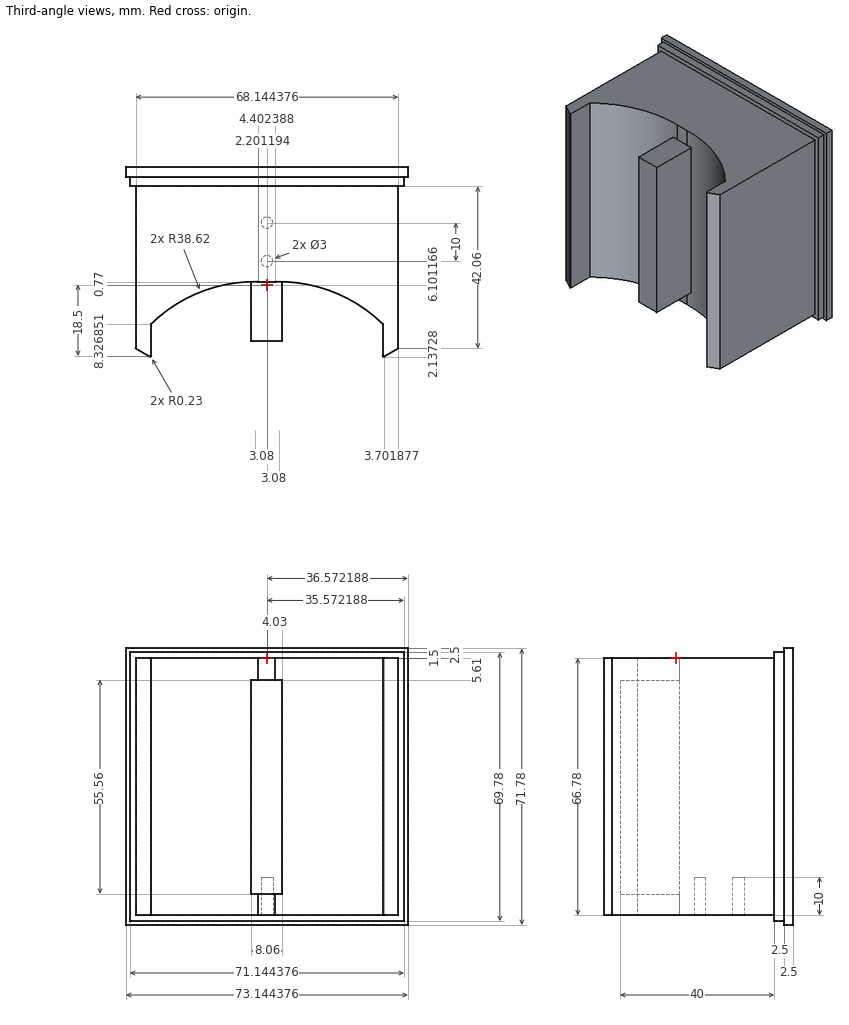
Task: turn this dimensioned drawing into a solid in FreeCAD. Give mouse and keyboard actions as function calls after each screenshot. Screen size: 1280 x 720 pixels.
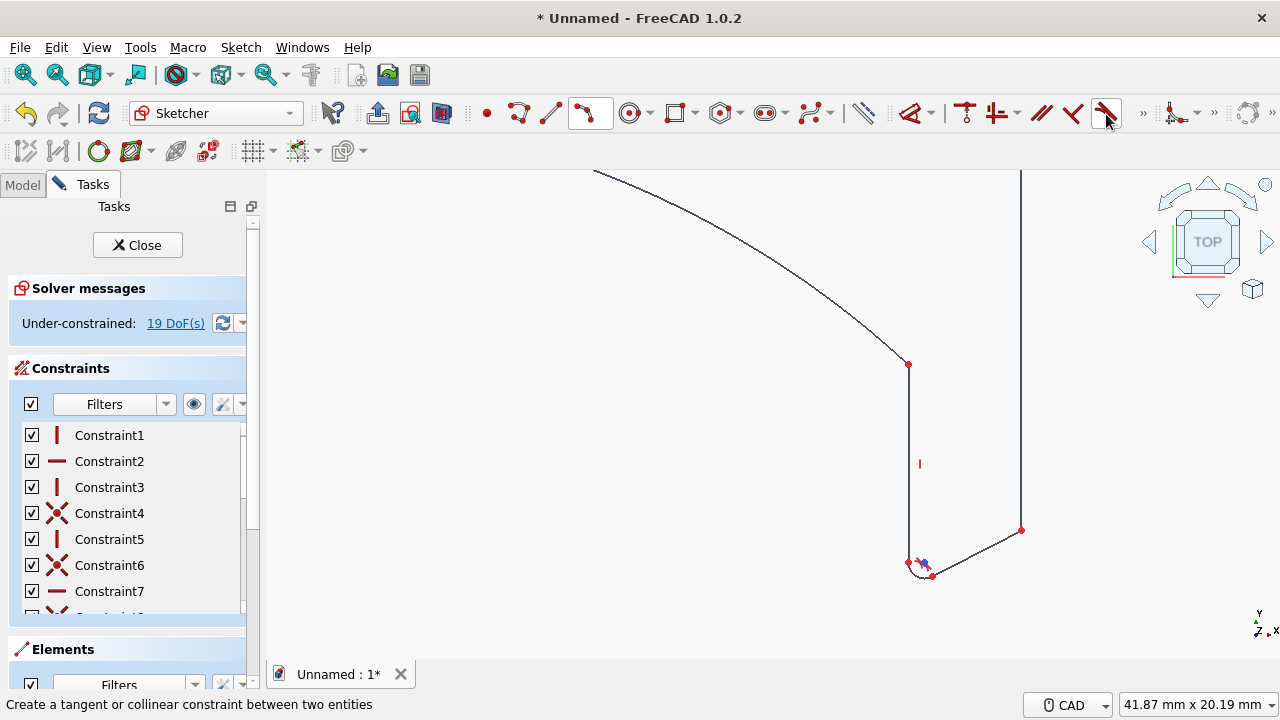
scroll(924, 575, down, 6)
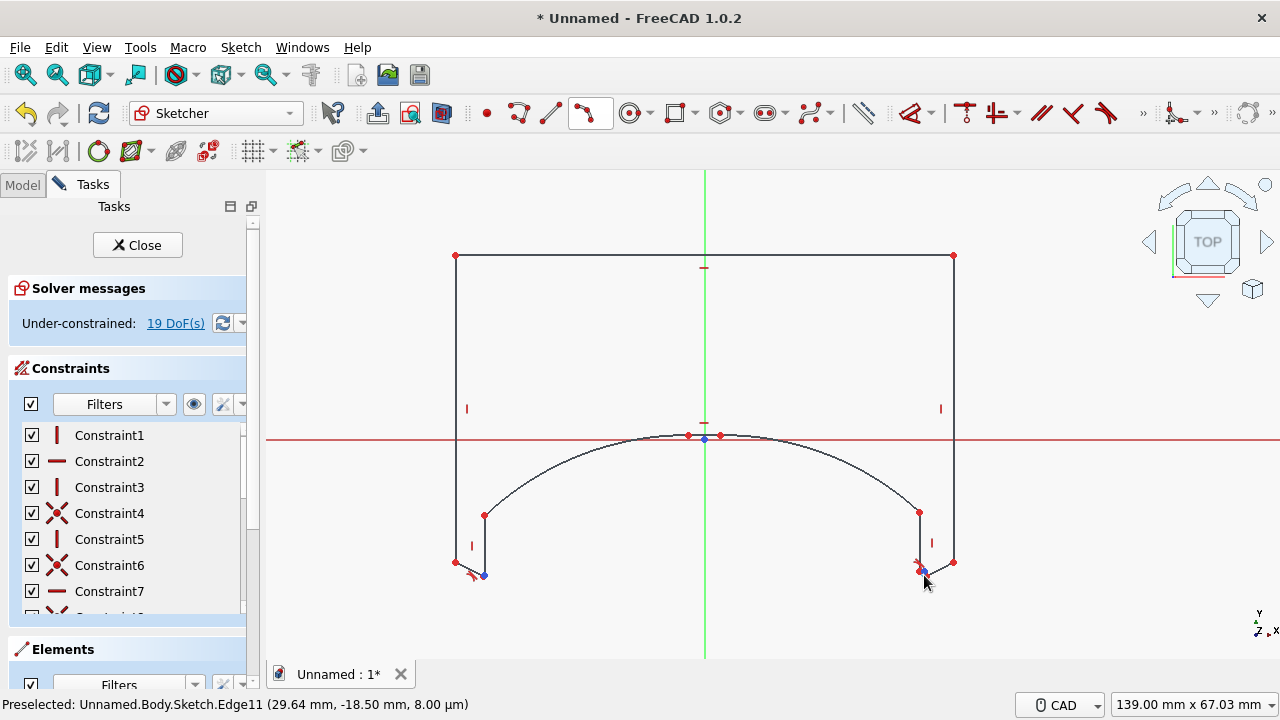
scroll(464, 566, up, 2)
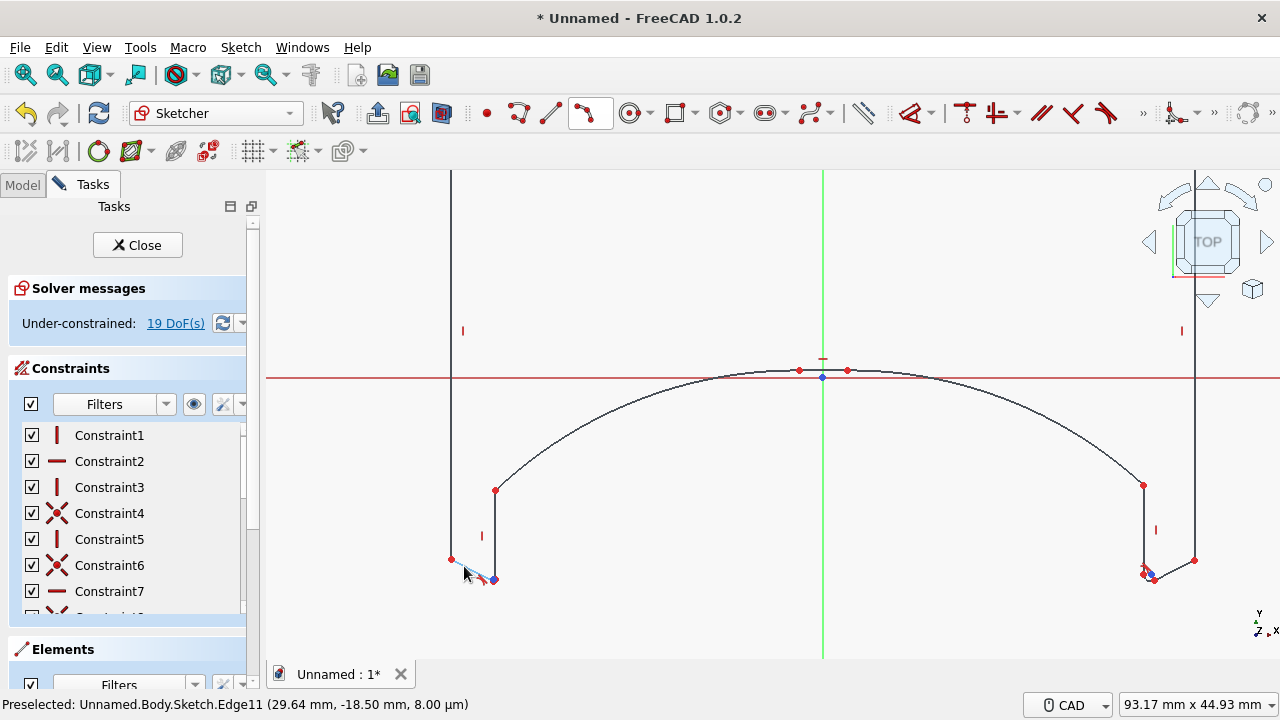
click(464, 566)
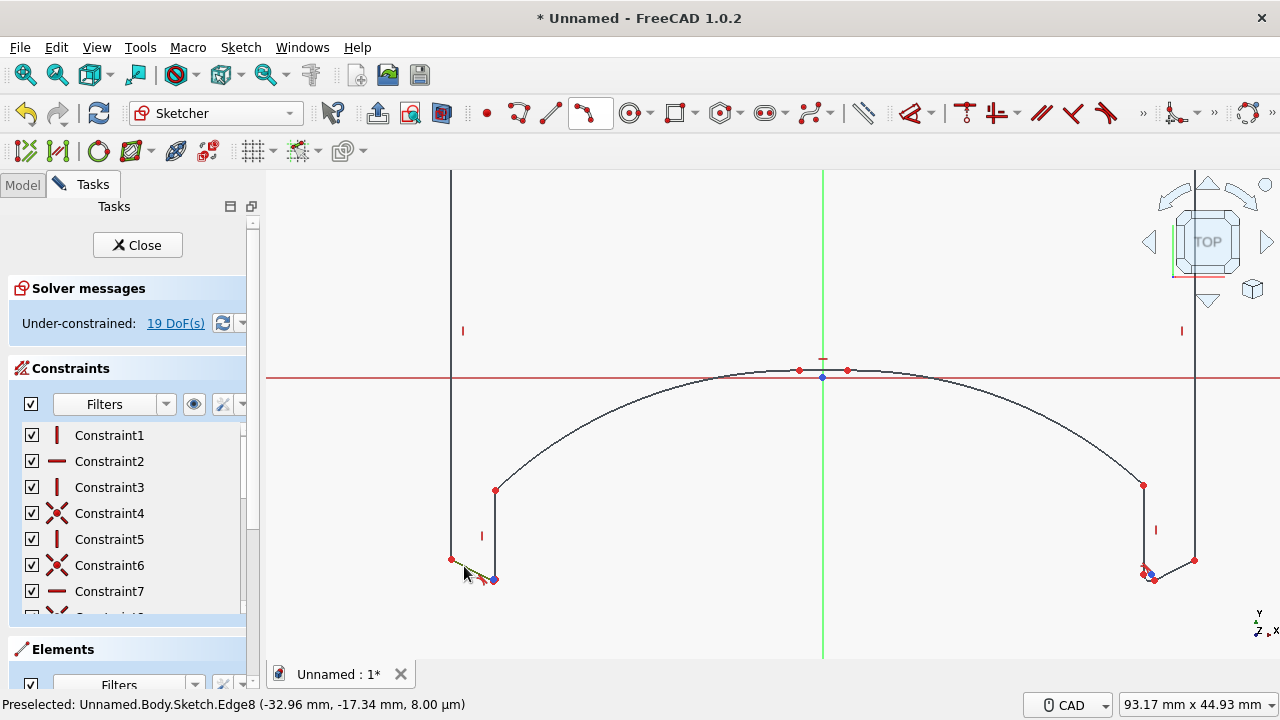
scroll(495, 581, up, 12)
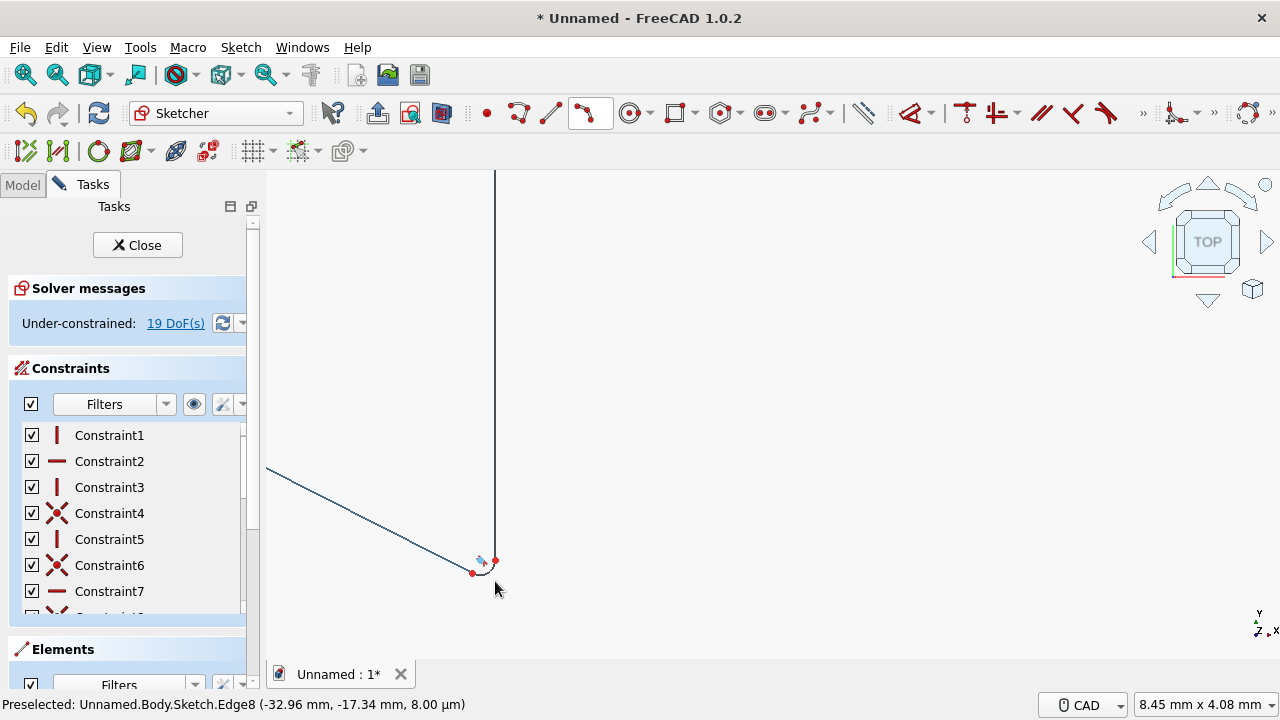
click(488, 573)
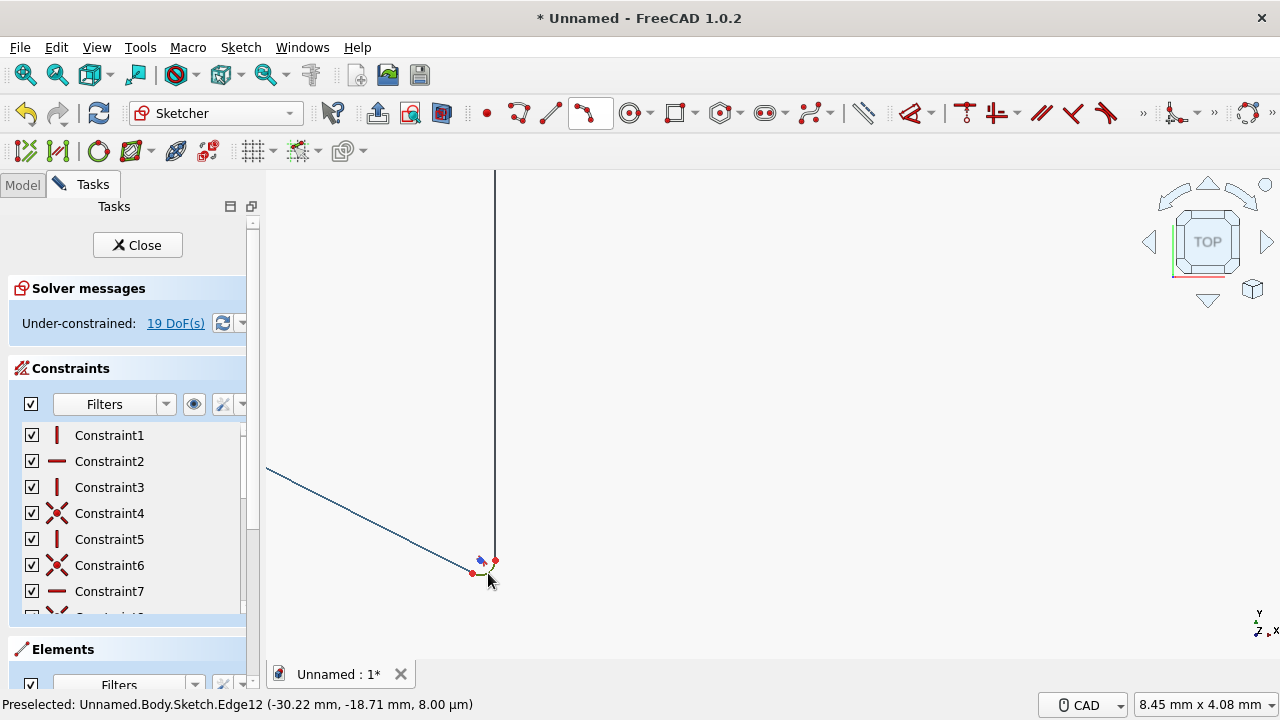
click(1106, 114)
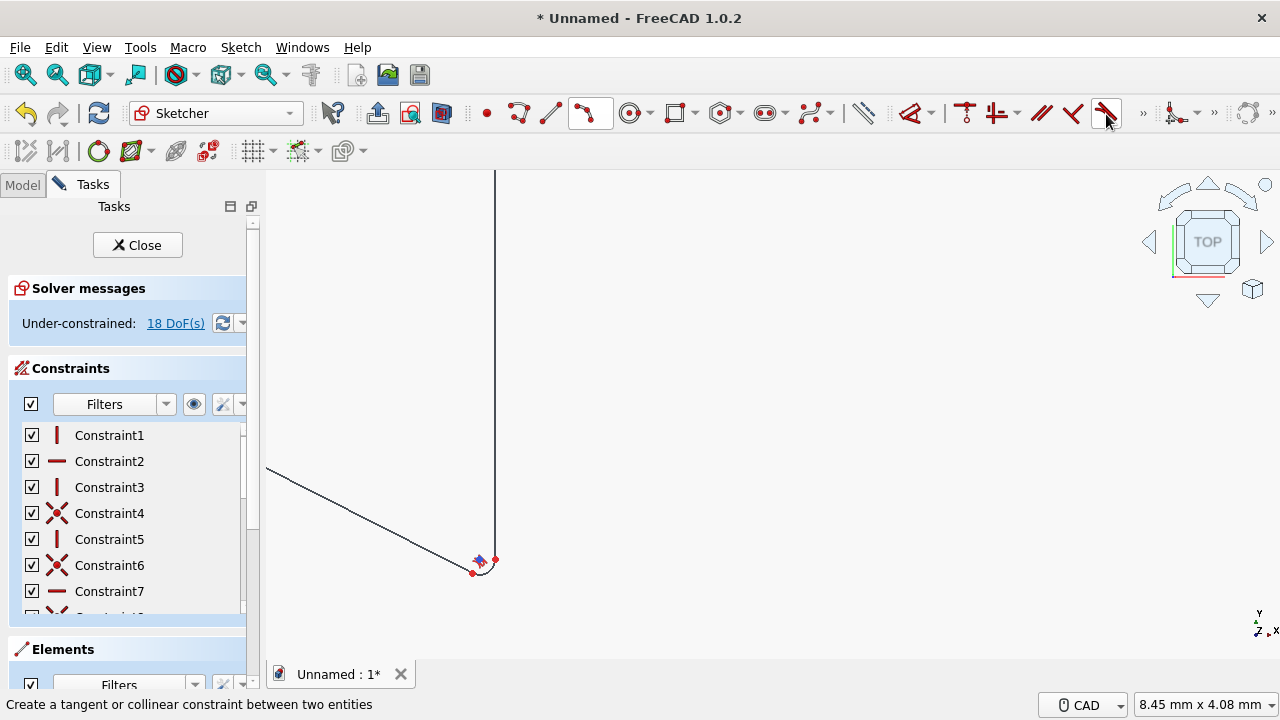
scroll(484, 576, down, 14)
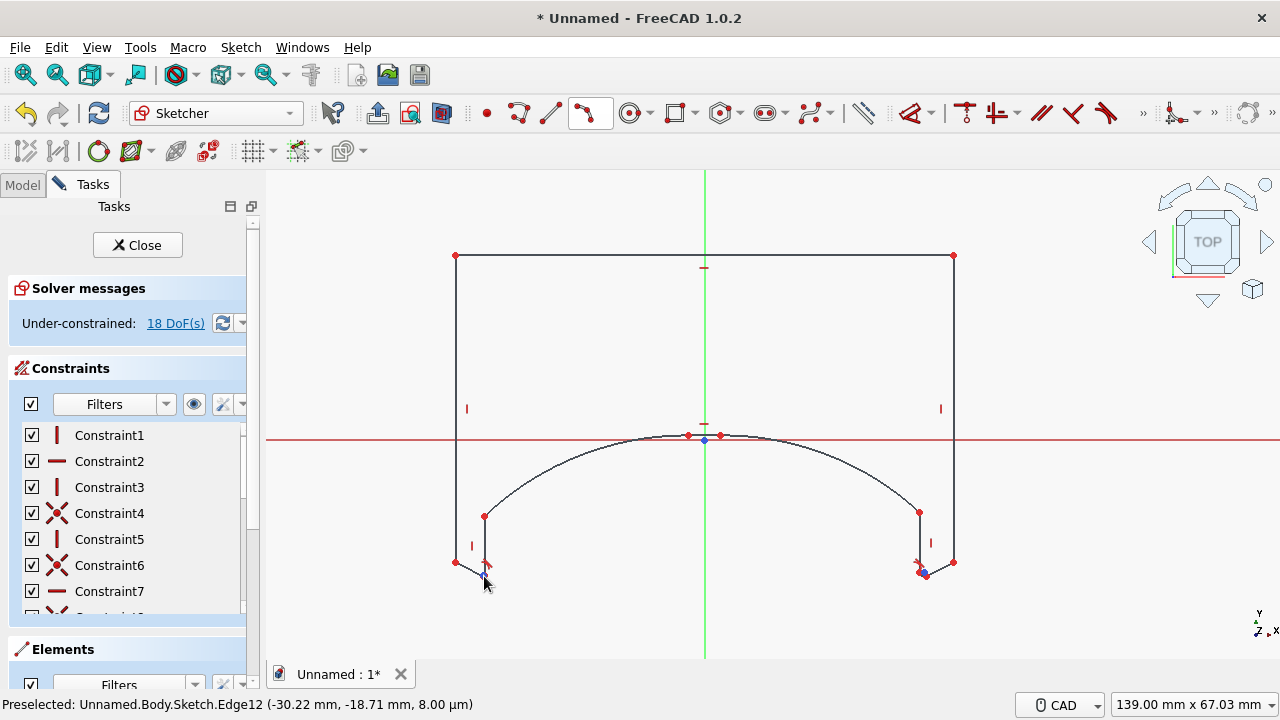
scroll(622, 443, up, 9)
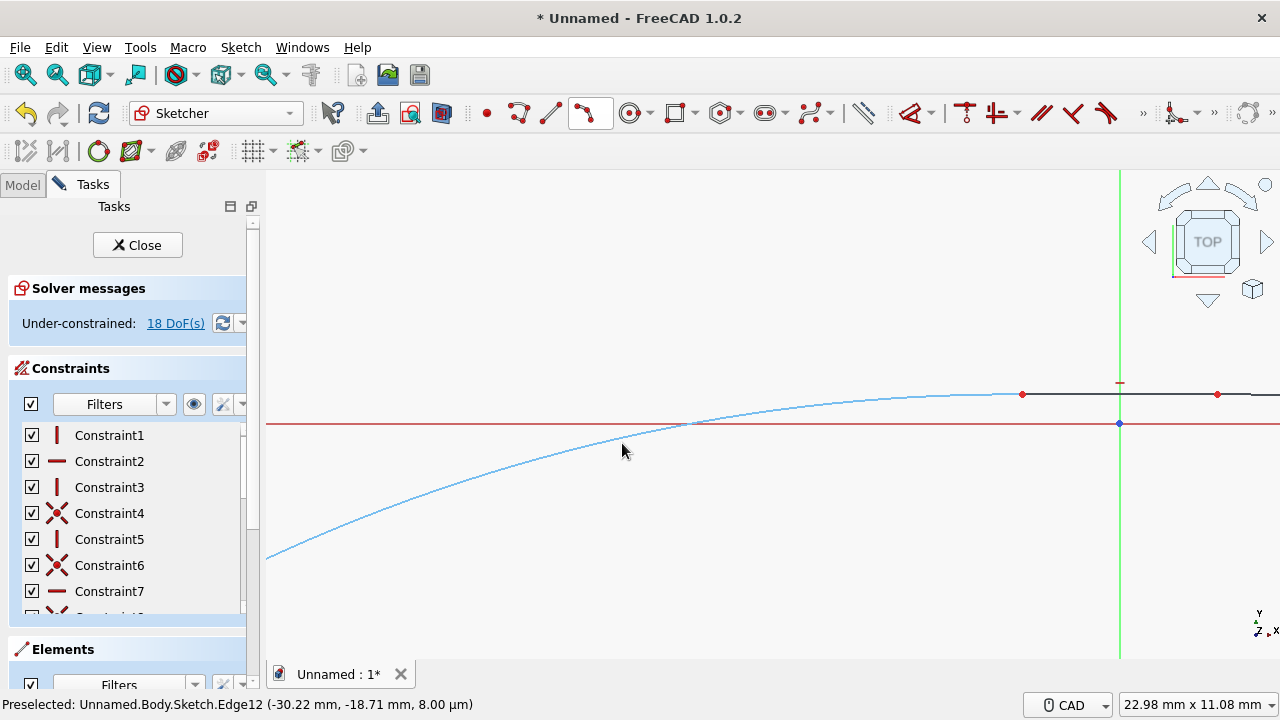
click(619, 439)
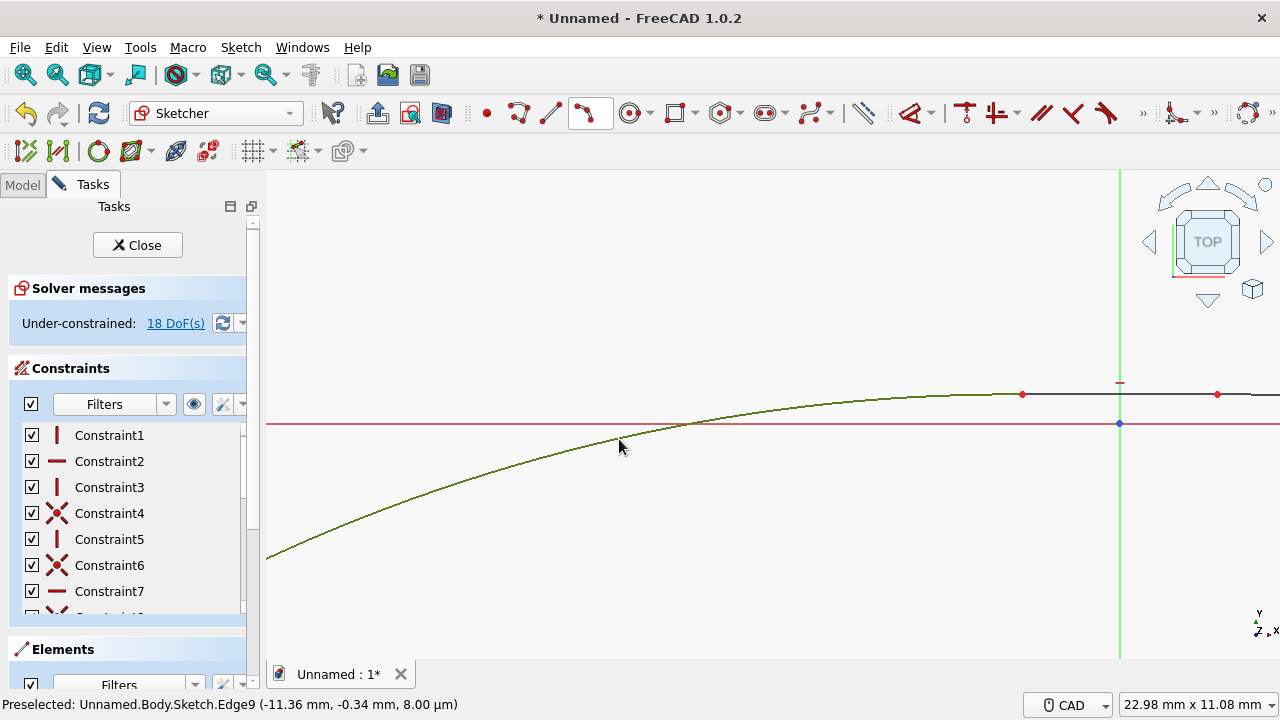
scroll(622, 442, down, 9)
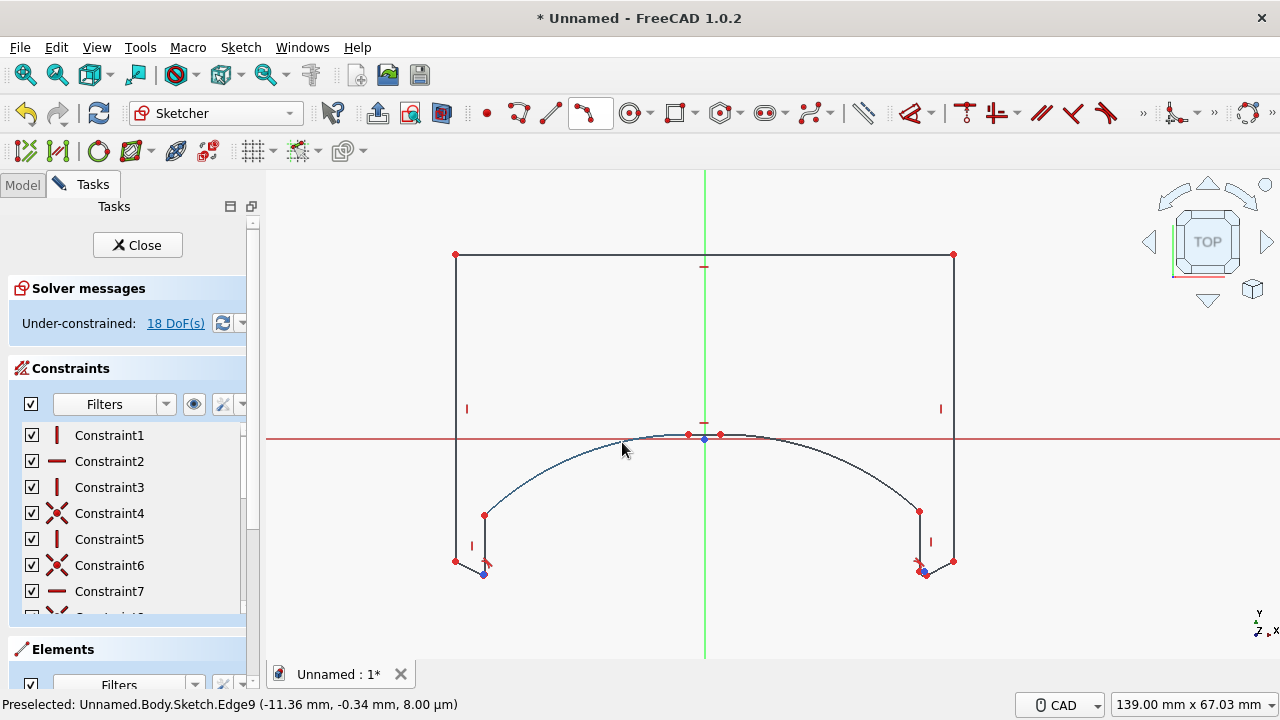
click(867, 473)